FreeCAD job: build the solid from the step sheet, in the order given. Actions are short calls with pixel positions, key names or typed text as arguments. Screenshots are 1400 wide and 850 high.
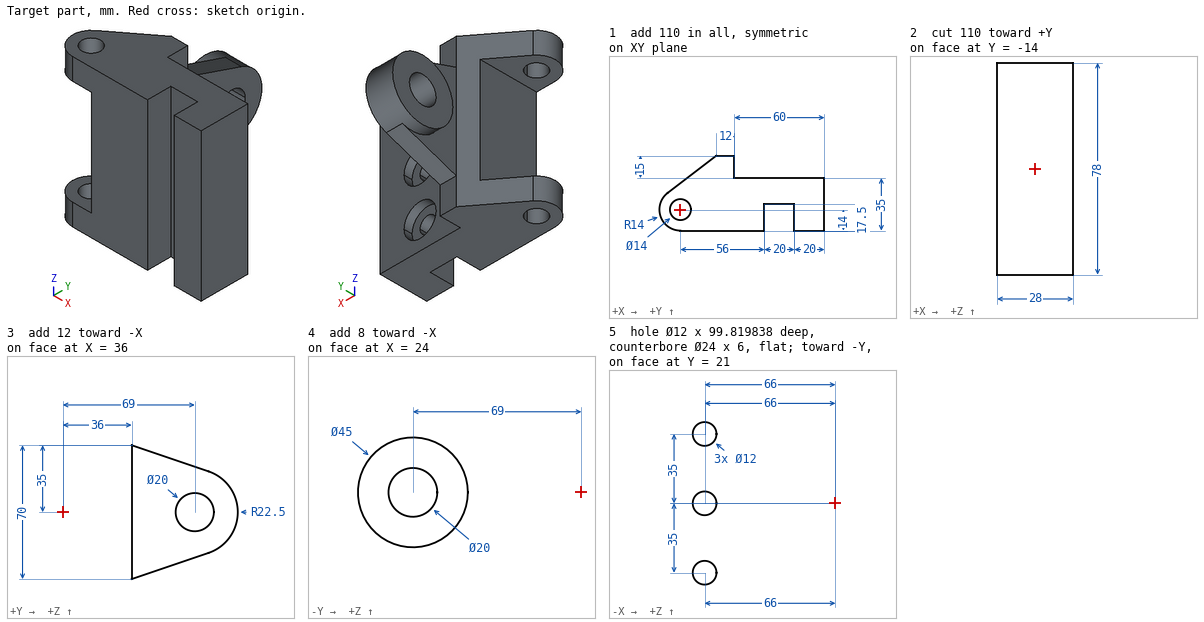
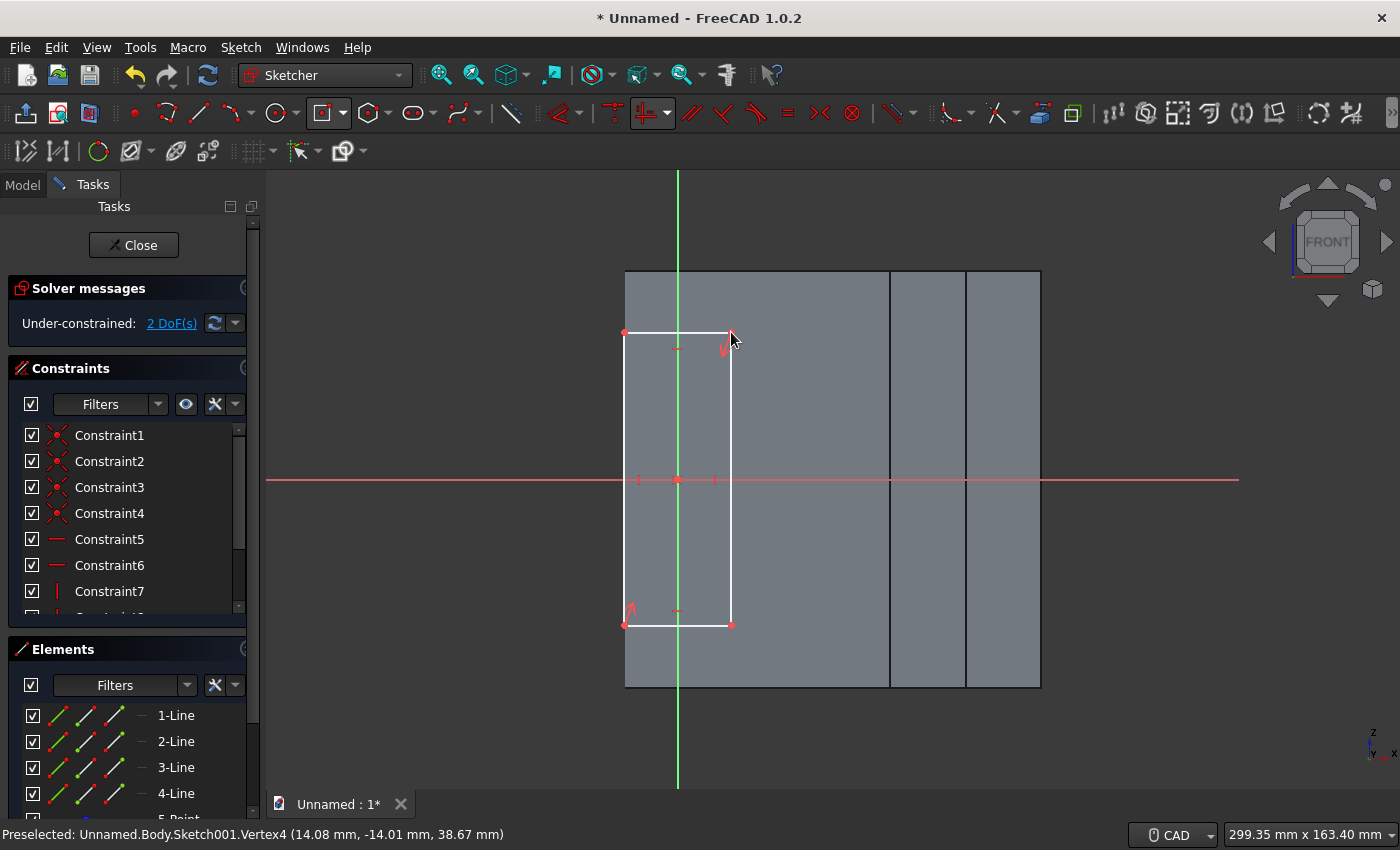
click(558, 114)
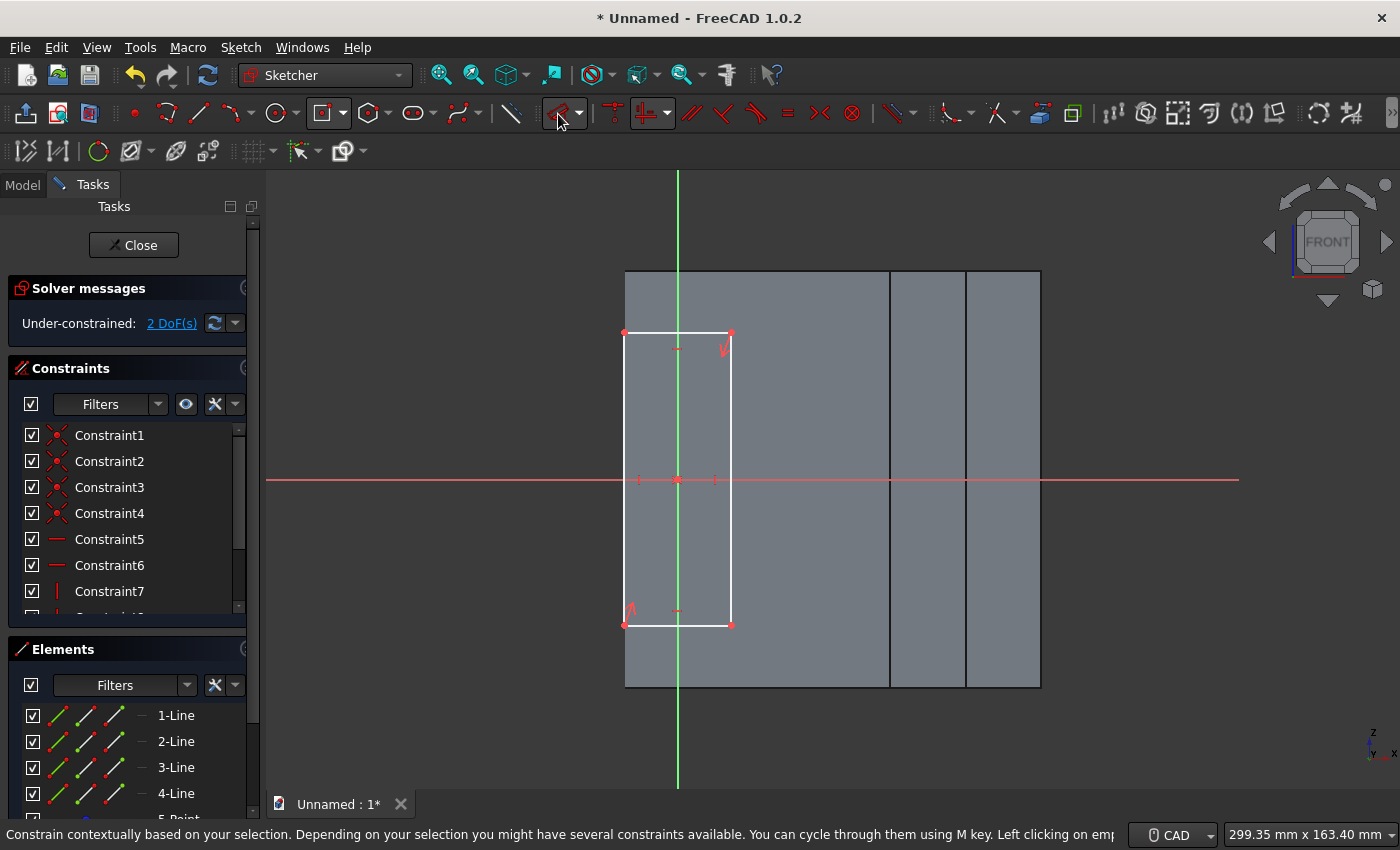
click(656, 626)
click(653, 660)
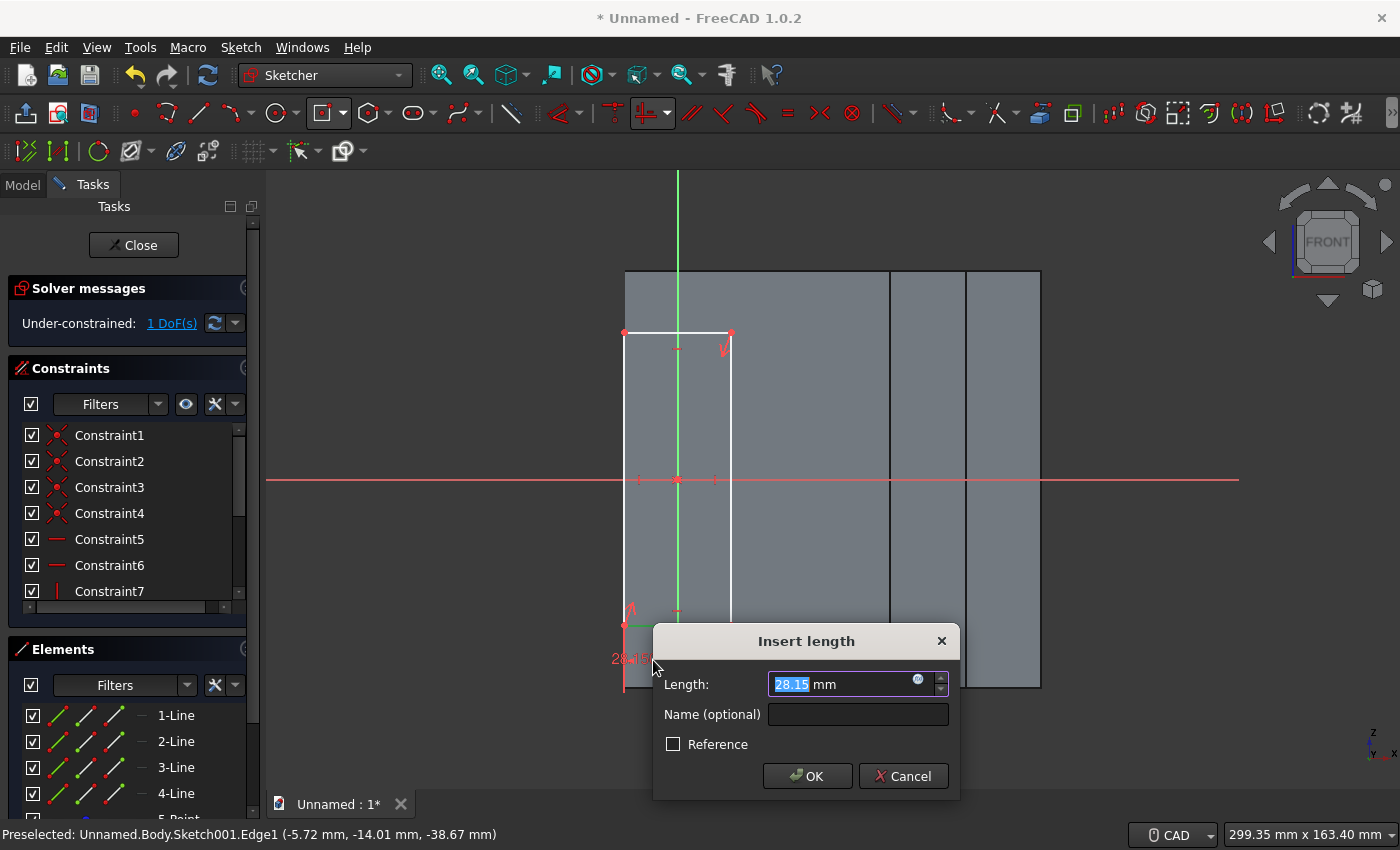
text(28)
key(Return)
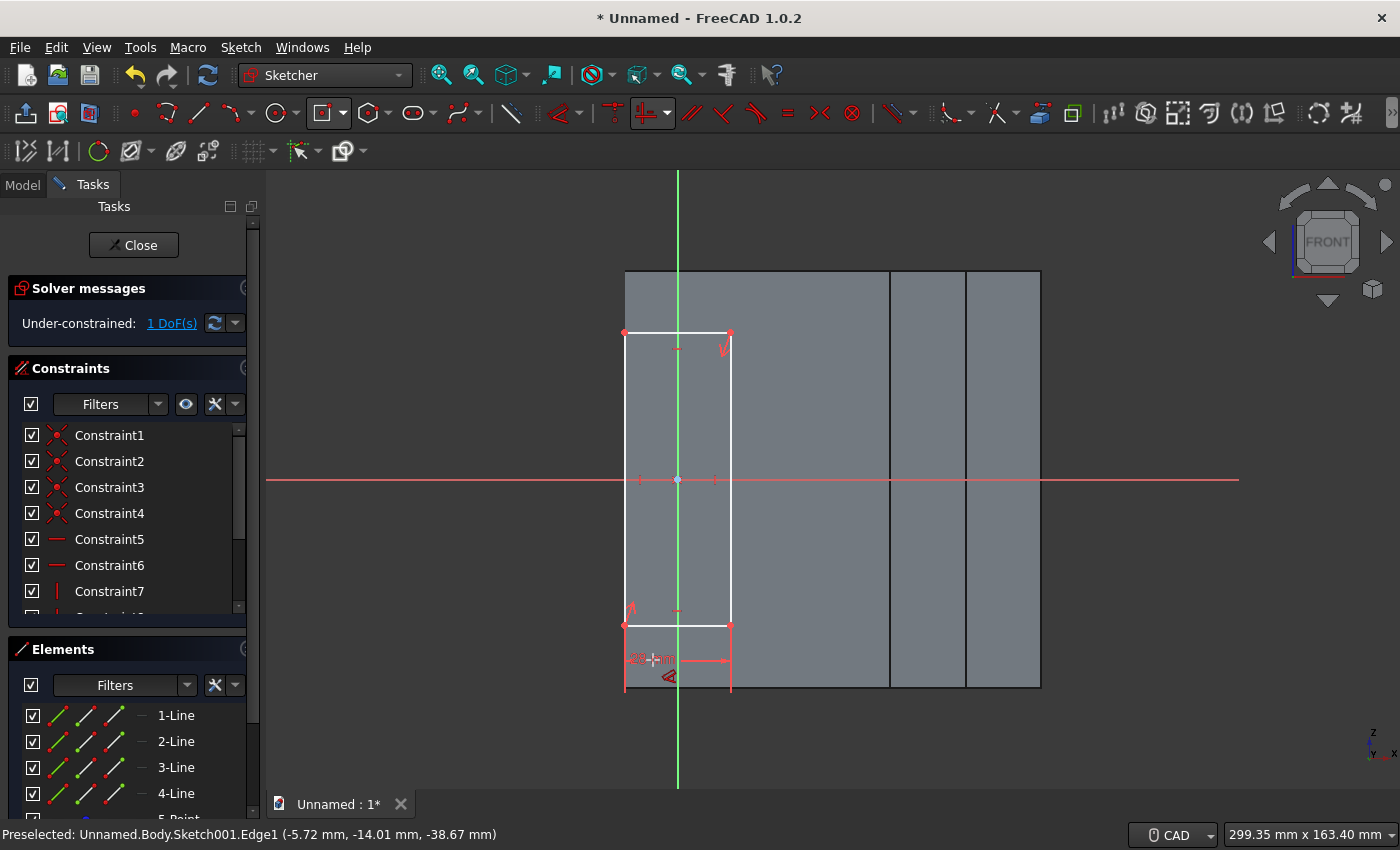
click(731, 538)
click(765, 412)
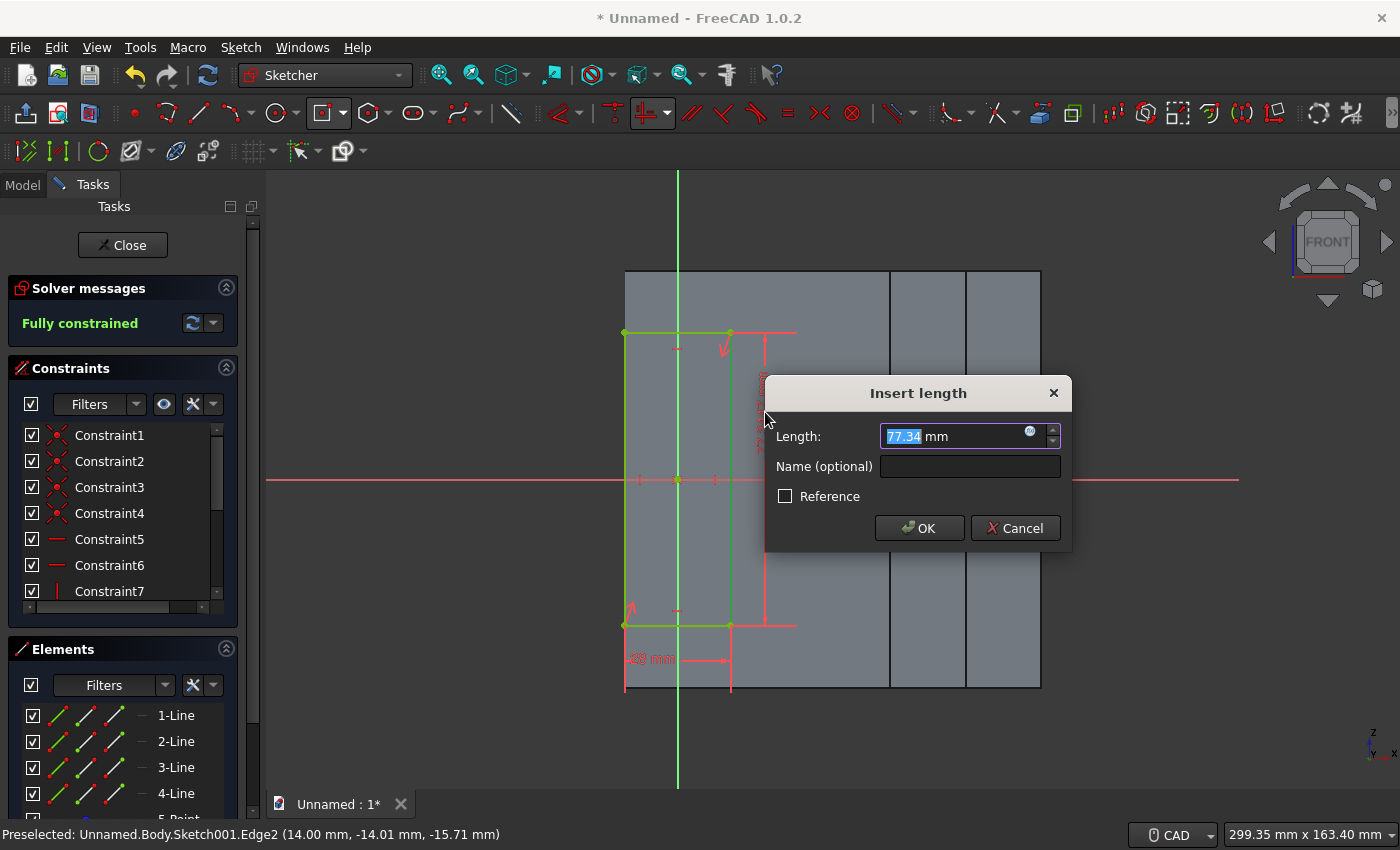
text(78)
key(Return)
key(Escape)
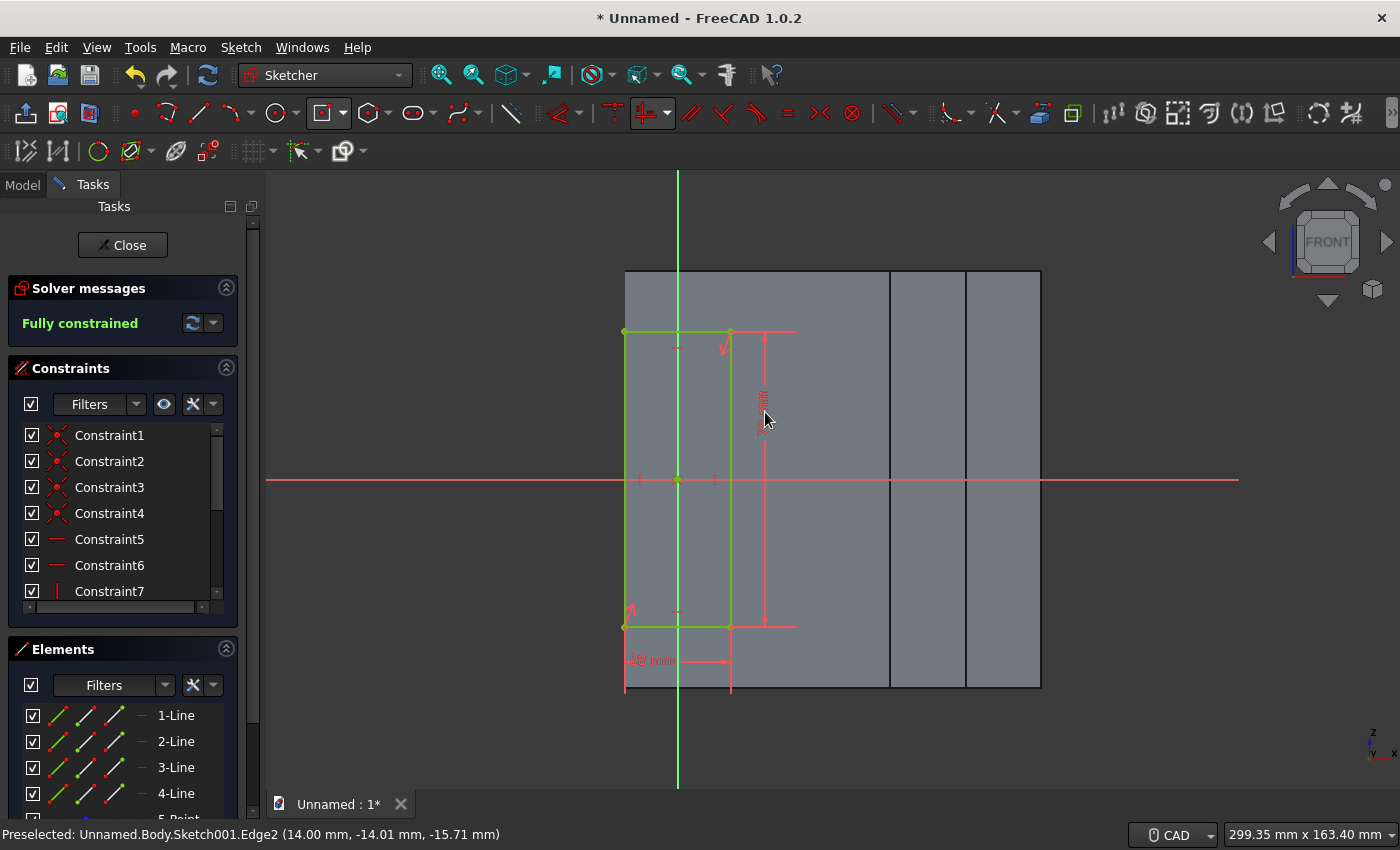
click(123, 245)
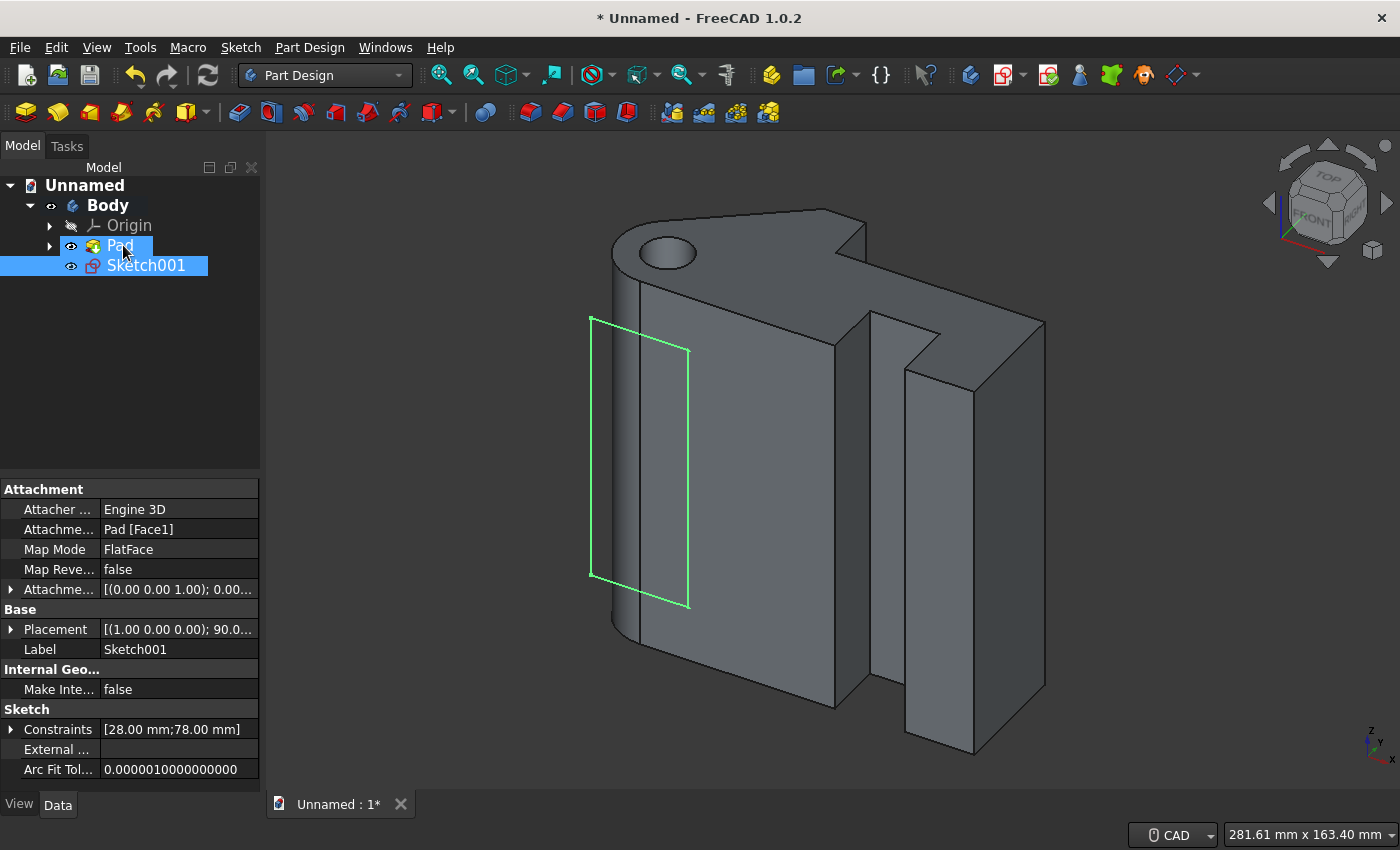
click(240, 112)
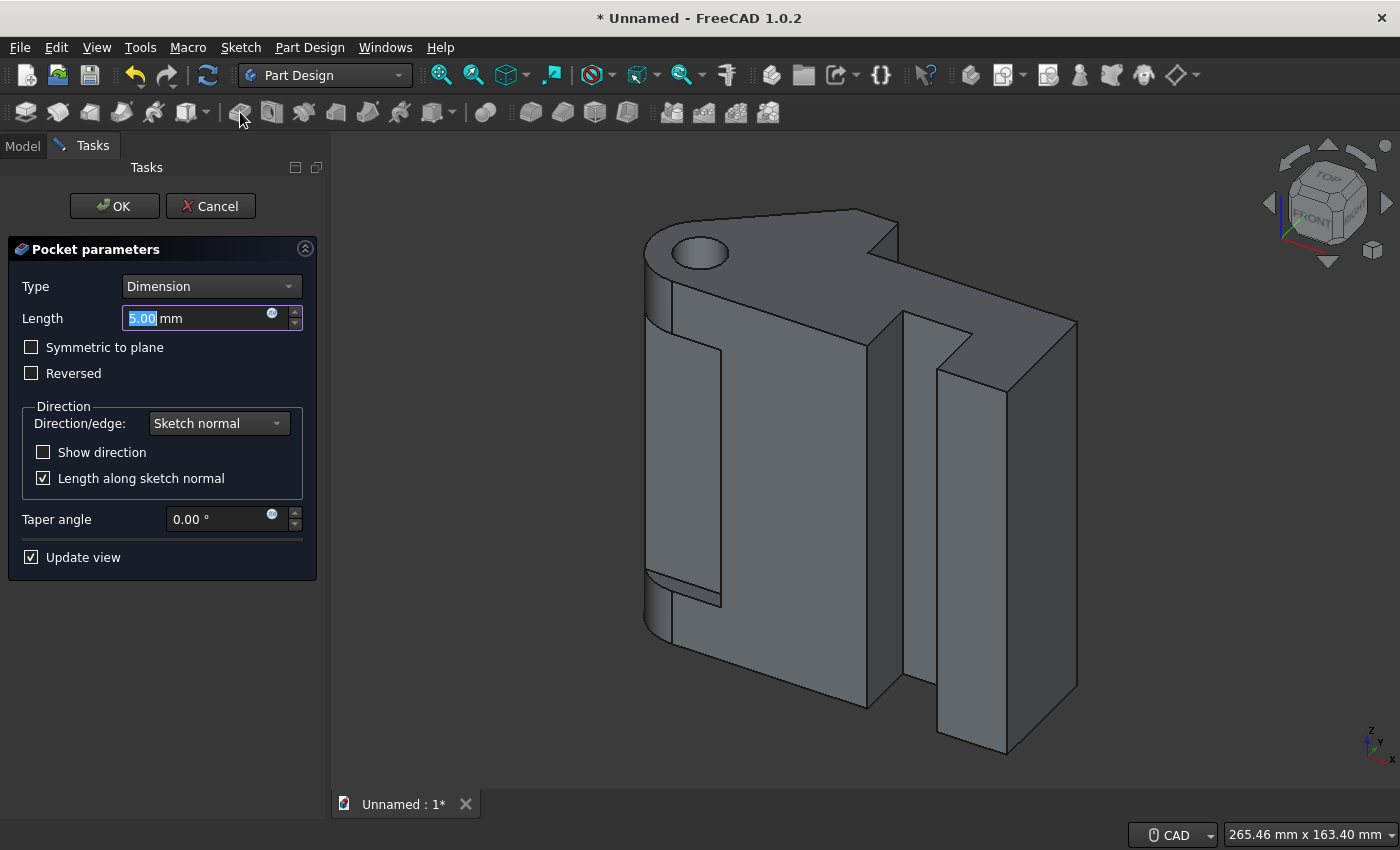
text(110)
key(Tab)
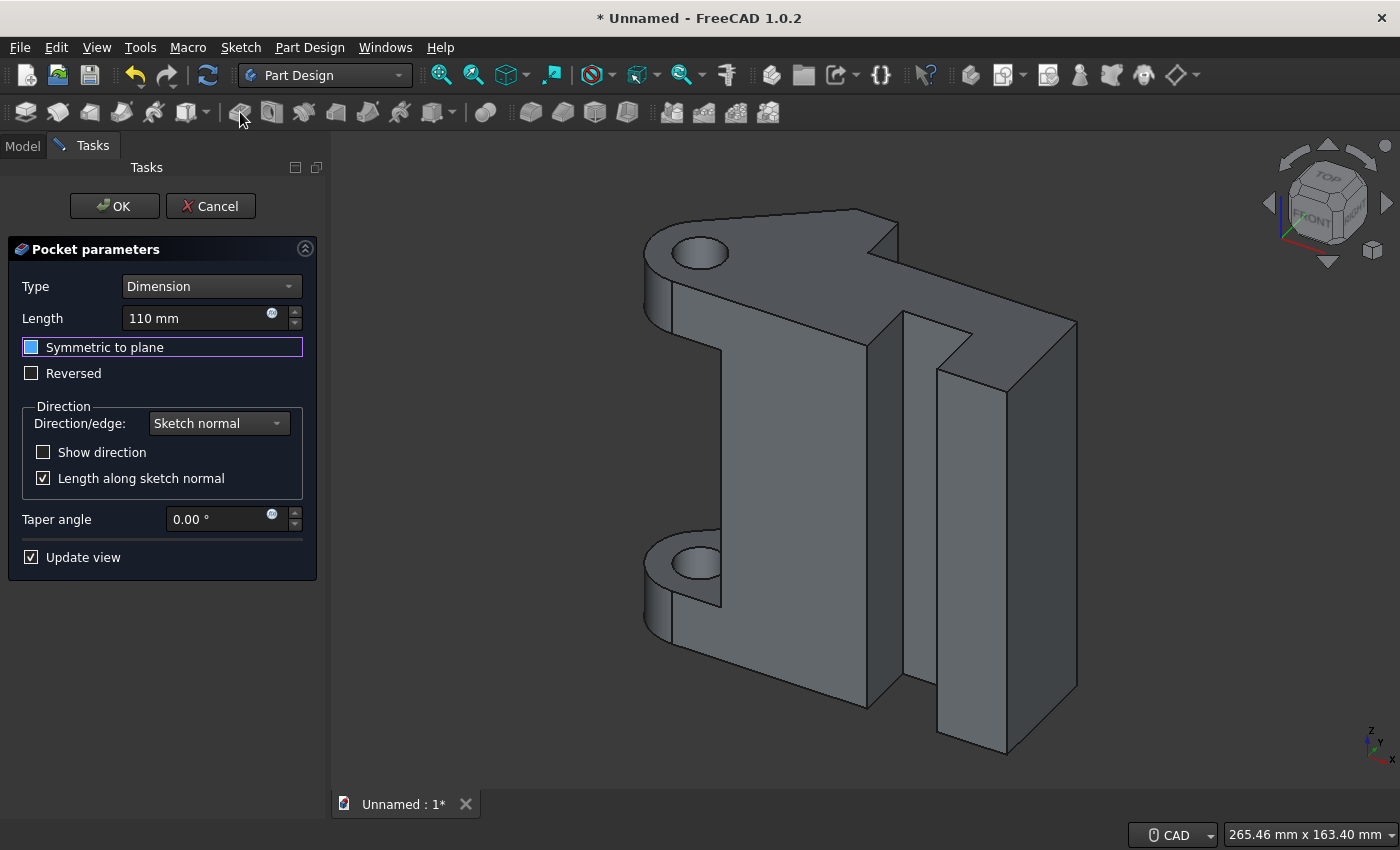
click(115, 206)